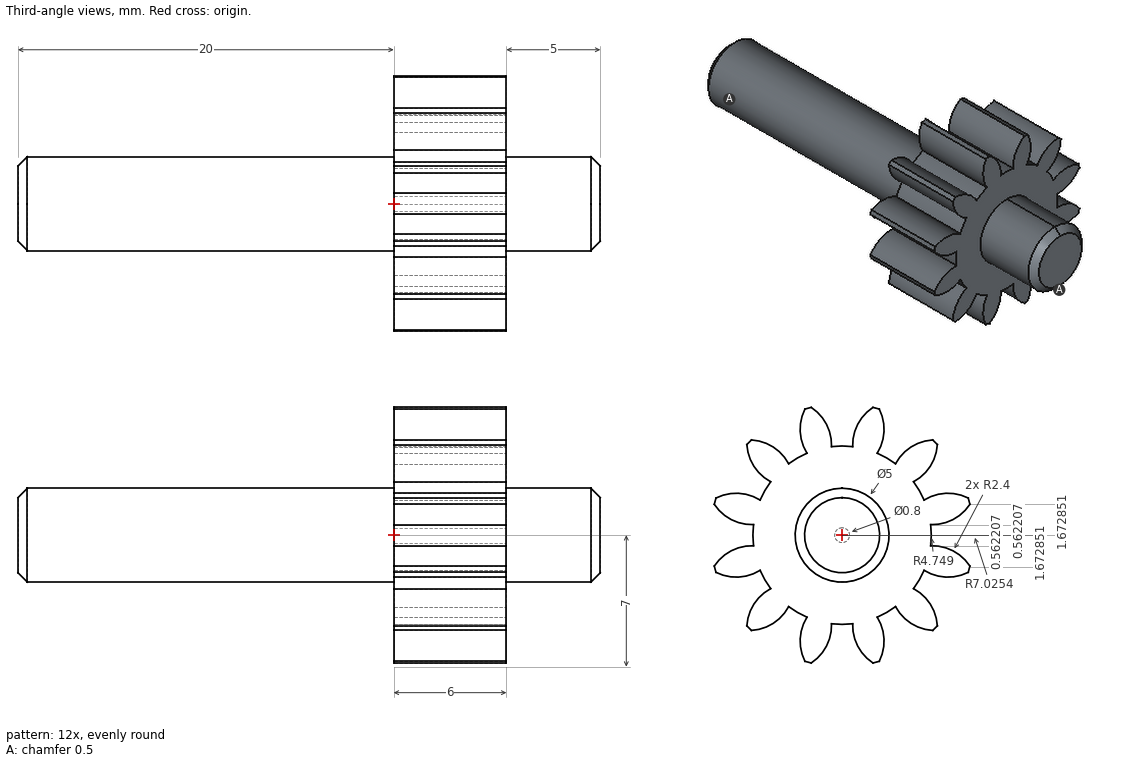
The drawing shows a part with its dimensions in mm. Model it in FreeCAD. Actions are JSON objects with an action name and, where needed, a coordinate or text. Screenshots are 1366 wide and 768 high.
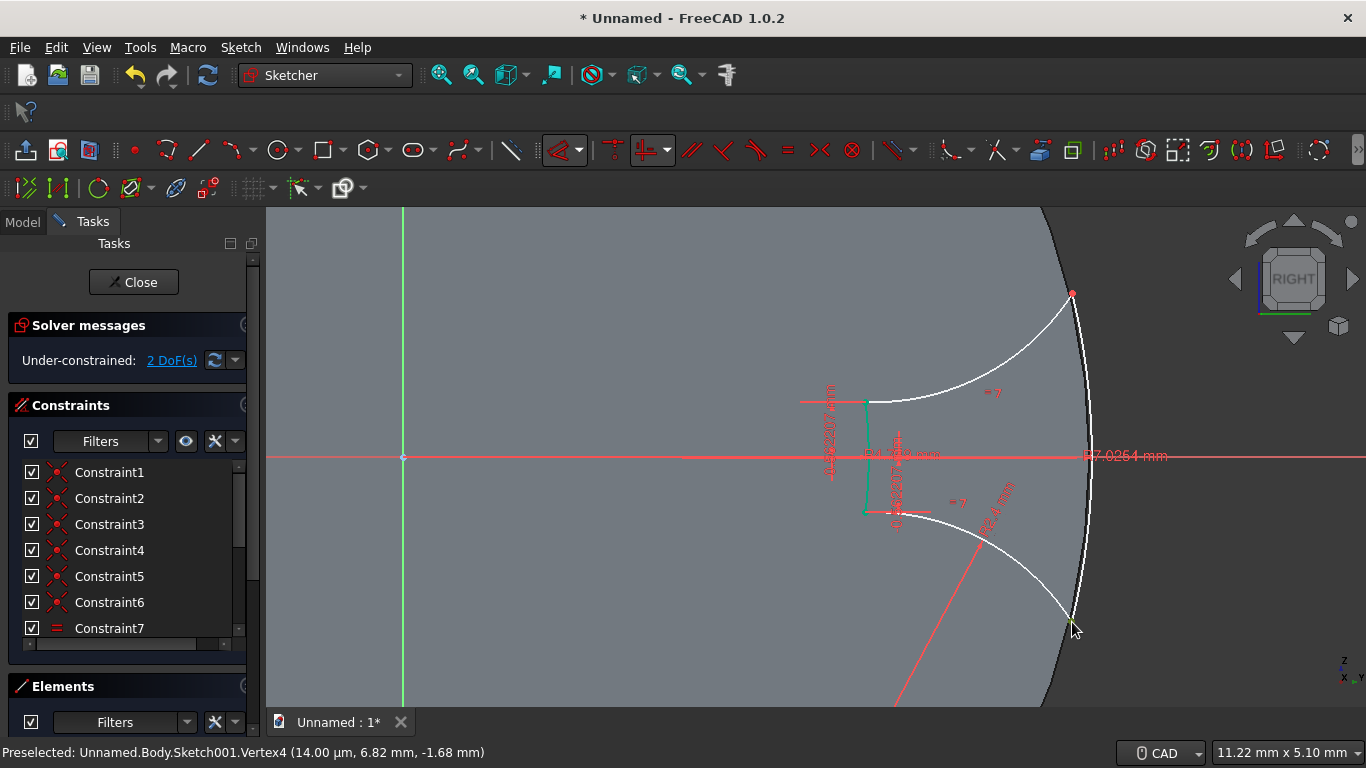
{"action": "left_click", "coordinate": [582, 150]}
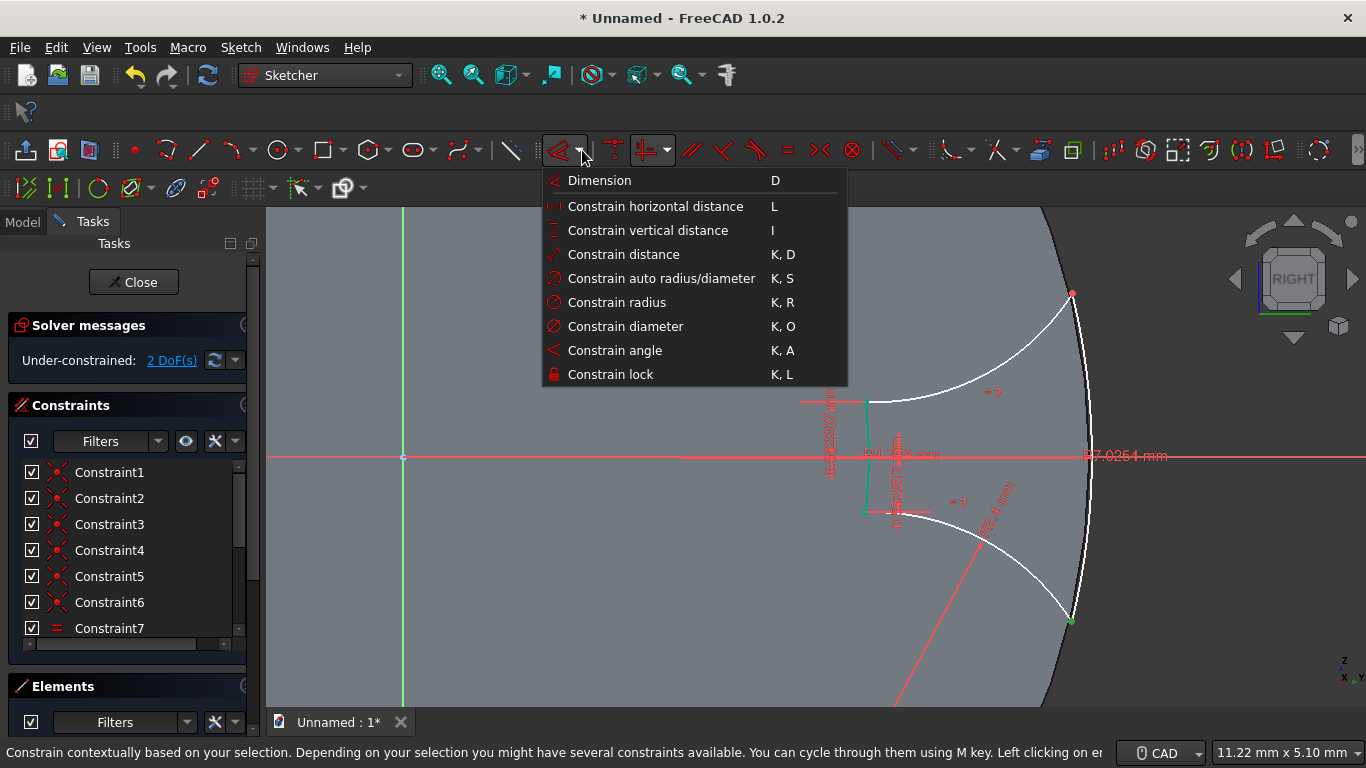
{"action": "left_click", "coordinate": [695, 230]}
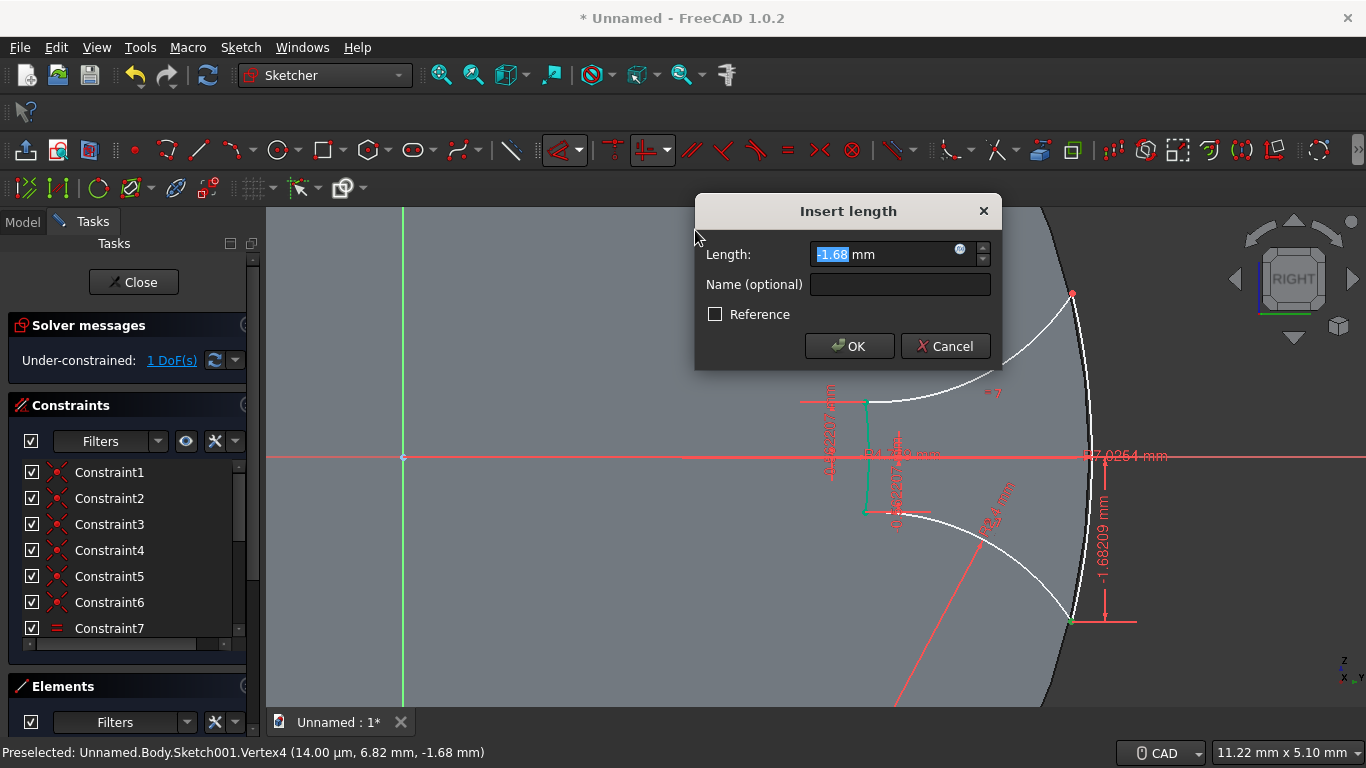
{"action": "type", "text": "-1.672851"}
{"action": "key", "text": "Return"}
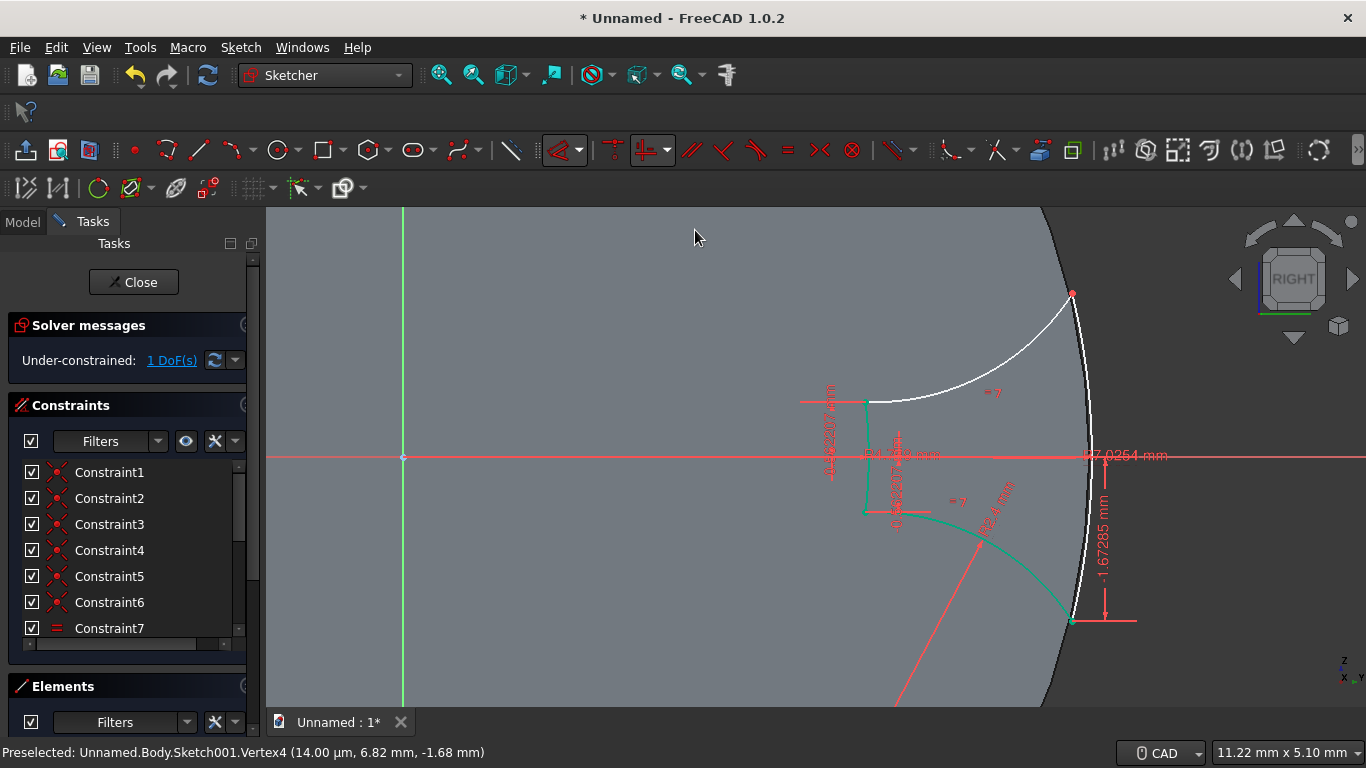
{"action": "left_click", "coordinate": [1072, 294]}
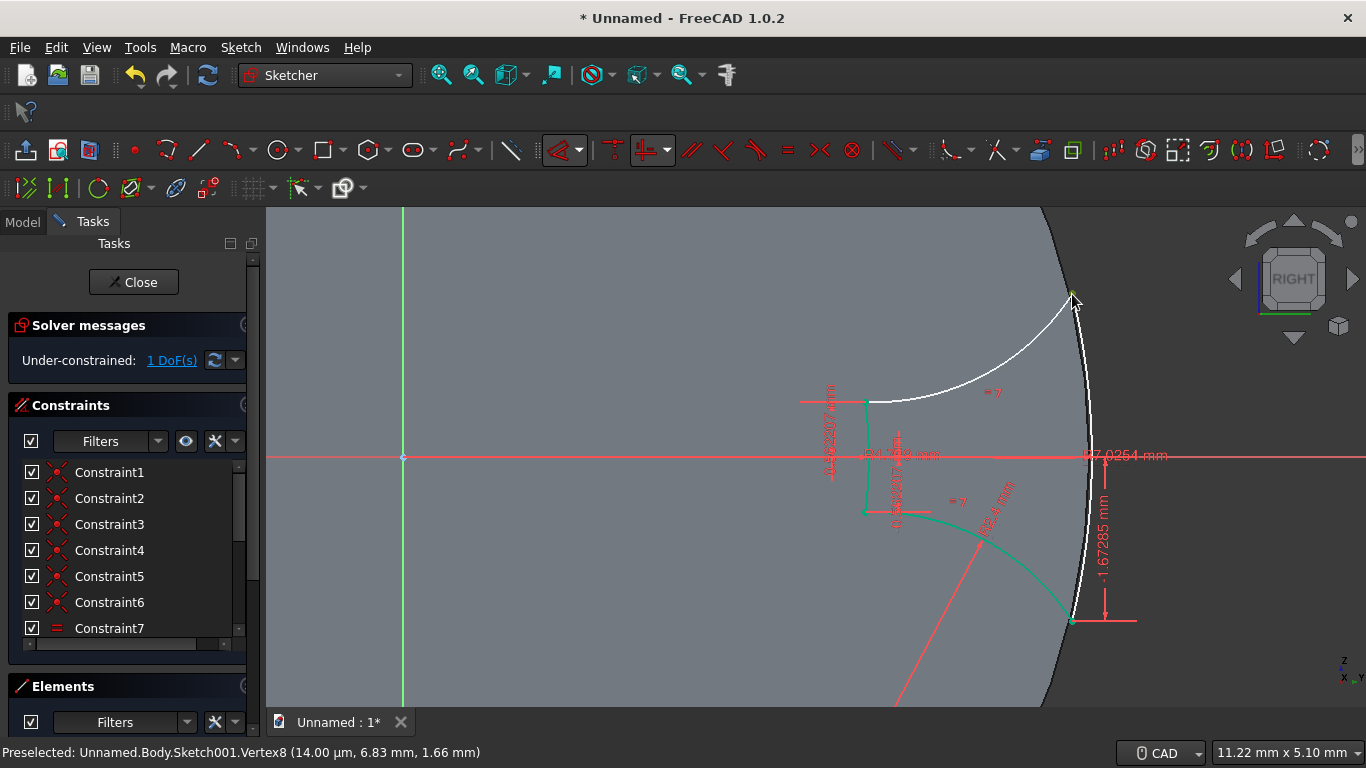
{"action": "left_click", "coordinate": [582, 150]}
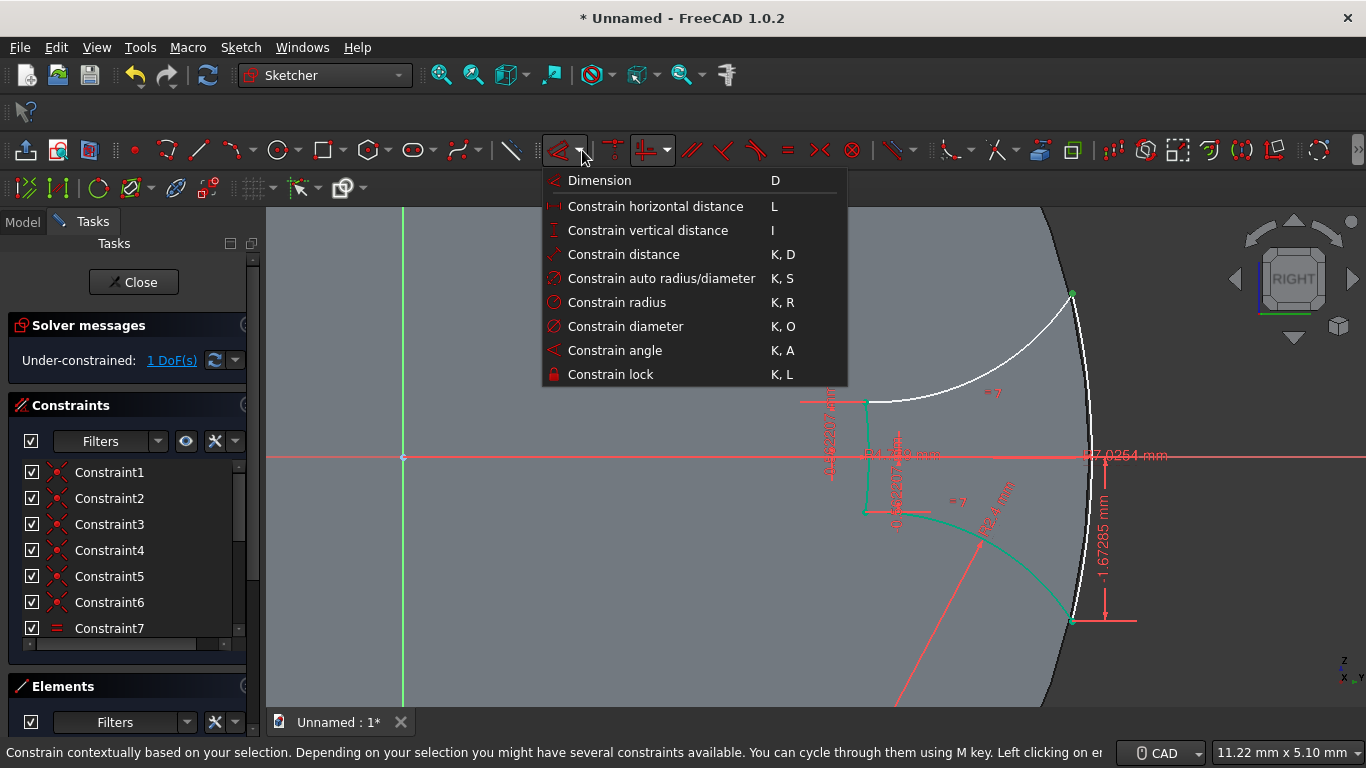
{"action": "left_click", "coordinate": [695, 230]}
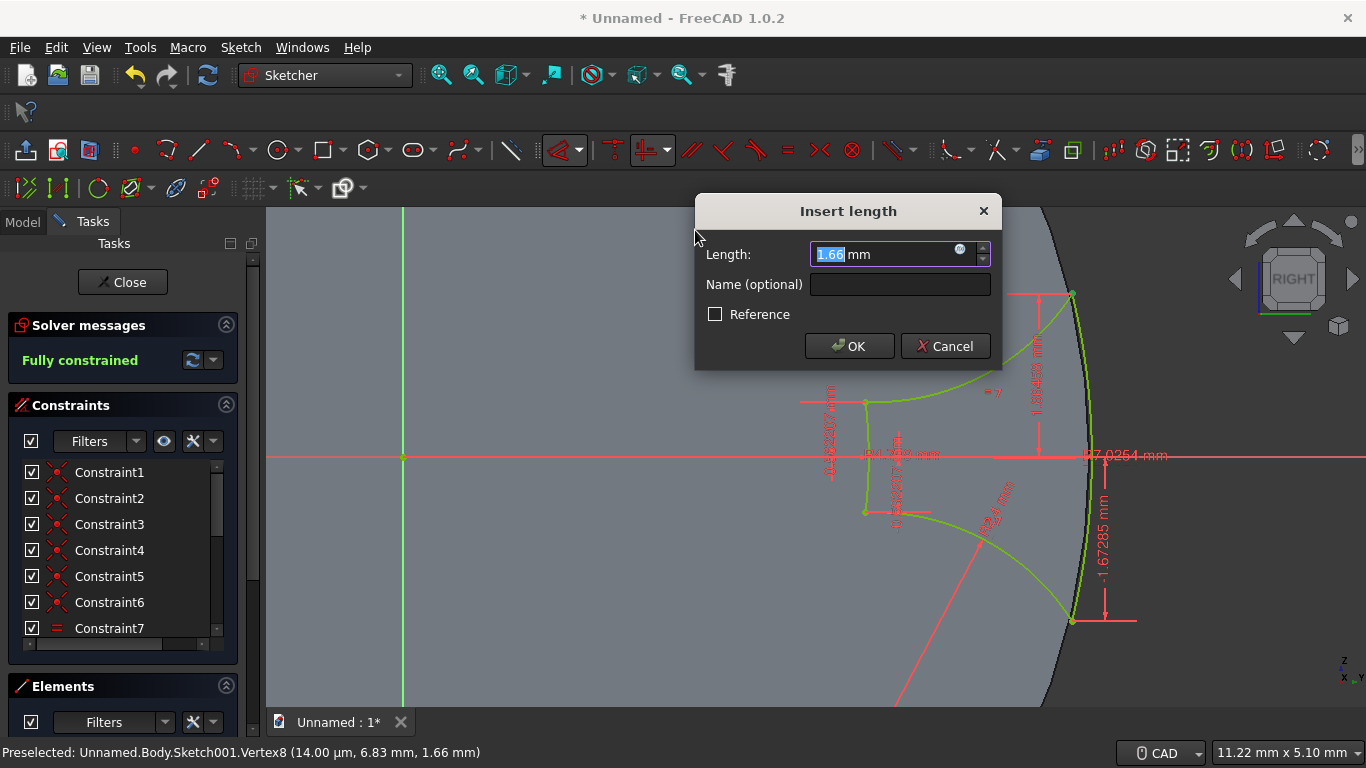
{"action": "type", "text": "1.672851"}
{"action": "key", "text": "Return"}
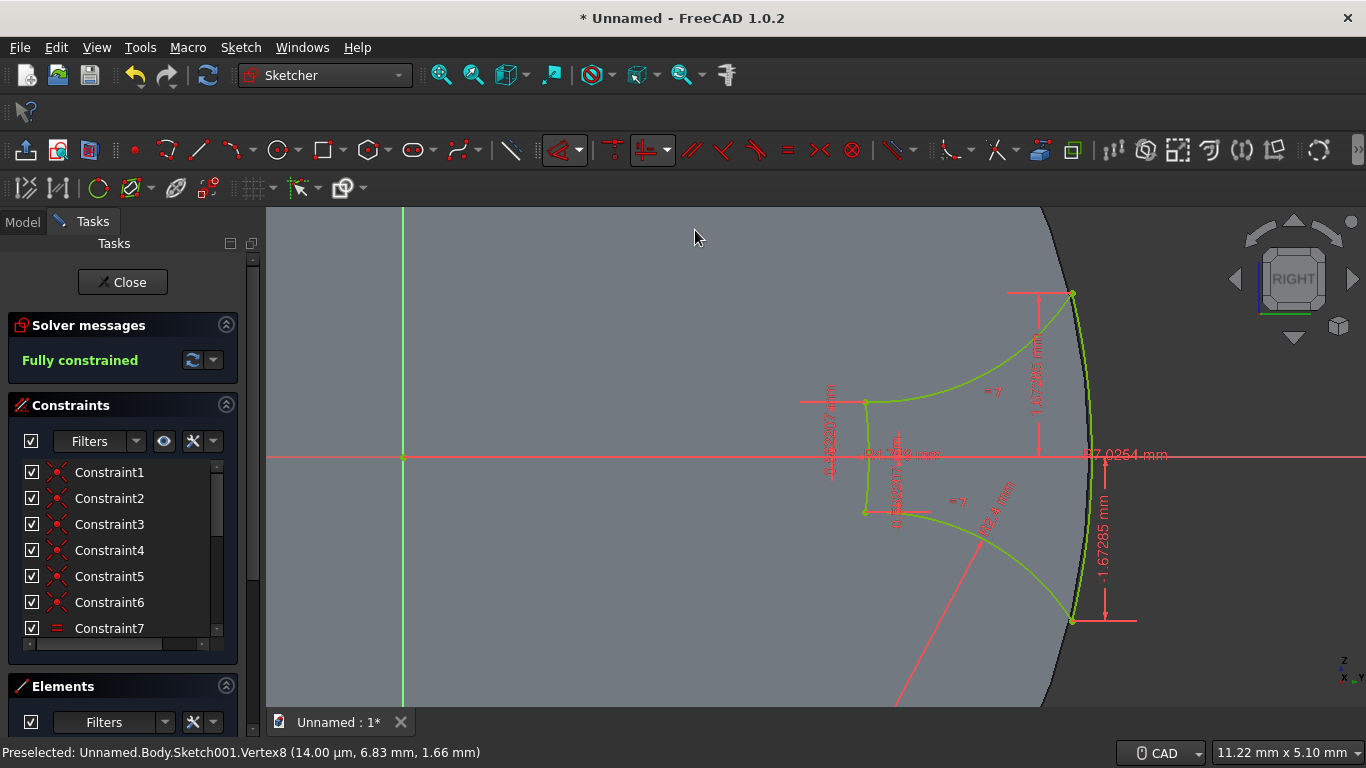
{"action": "left_click", "coordinate": [123, 282]}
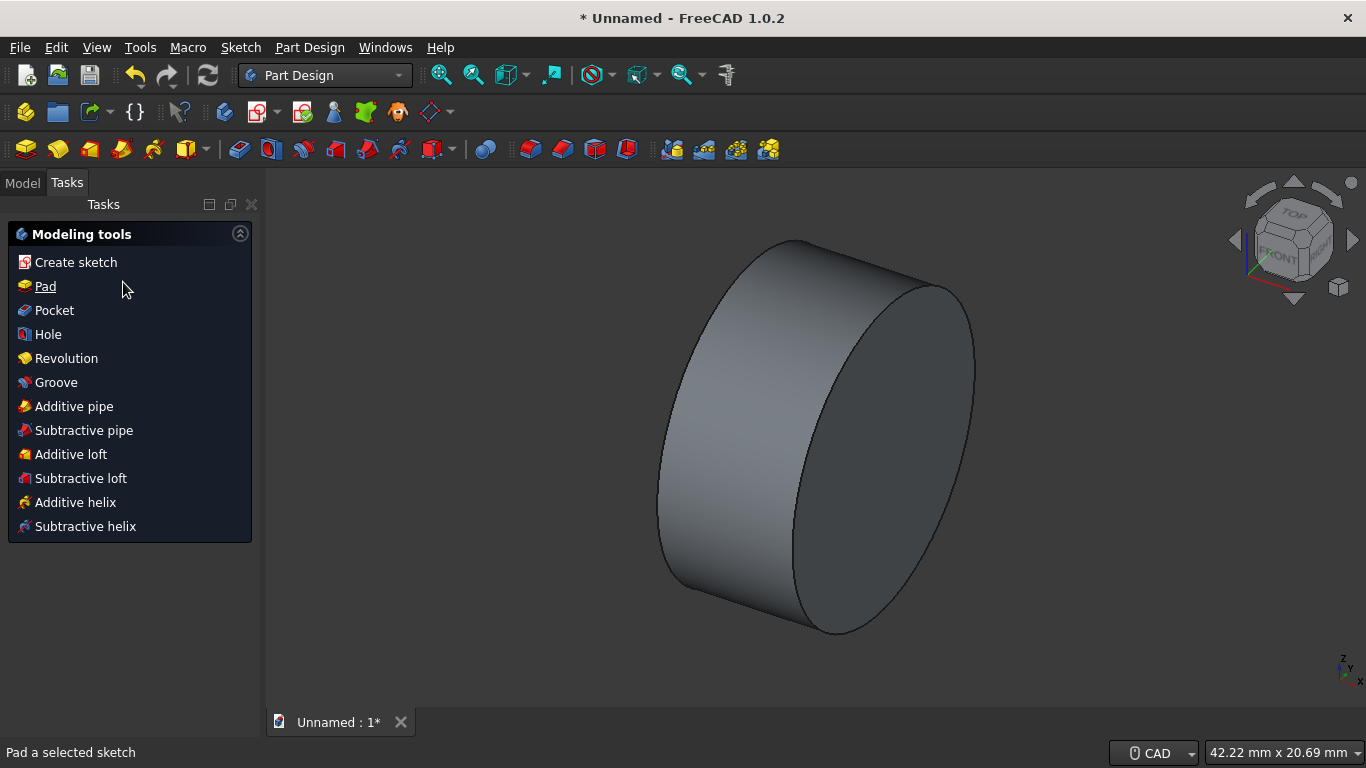
{"action": "left_click", "coordinate": [240, 150]}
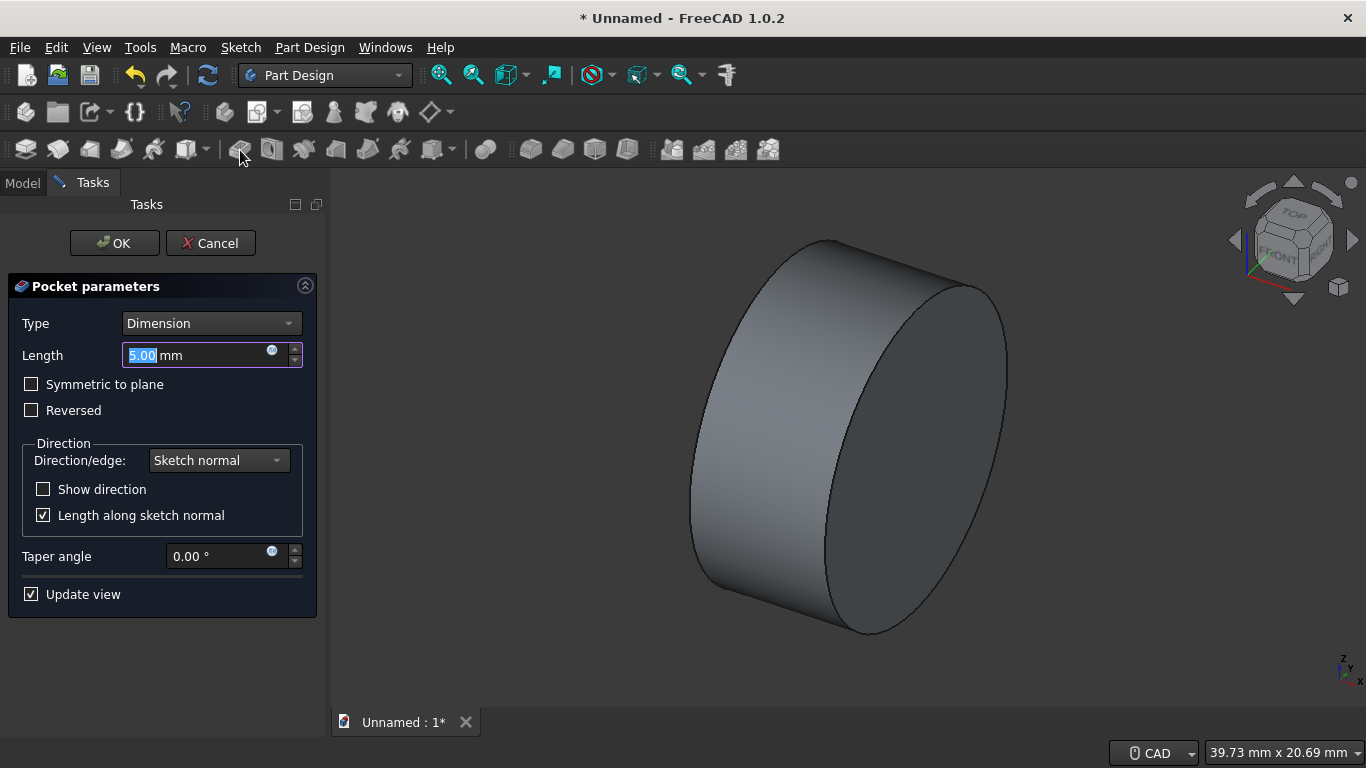
{"action": "left_click", "coordinate": [212, 324]}